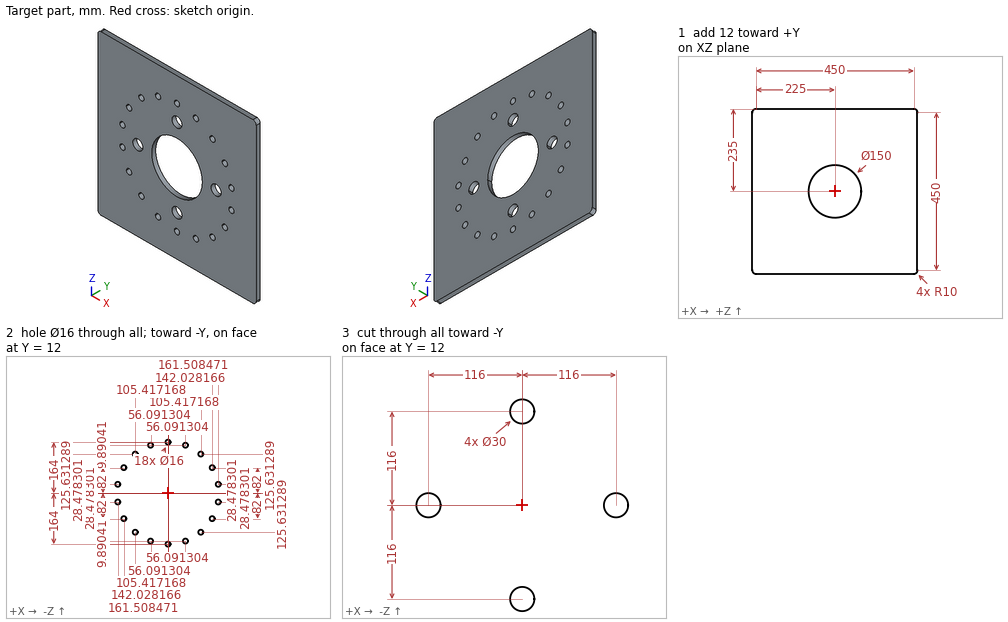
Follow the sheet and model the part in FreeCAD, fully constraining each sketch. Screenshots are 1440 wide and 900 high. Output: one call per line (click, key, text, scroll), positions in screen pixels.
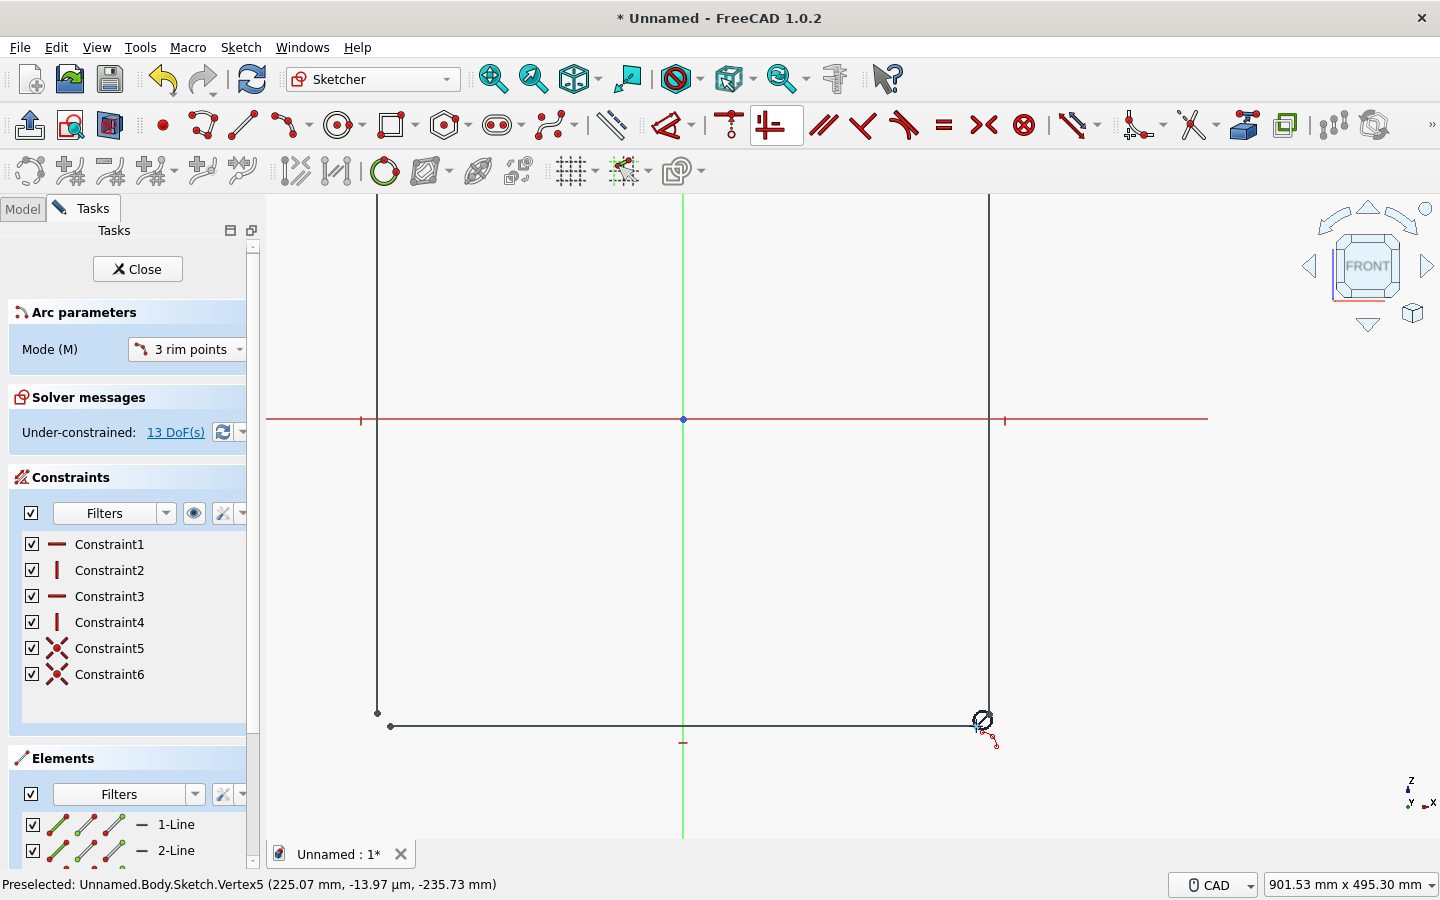
scroll(985, 722, up, 8)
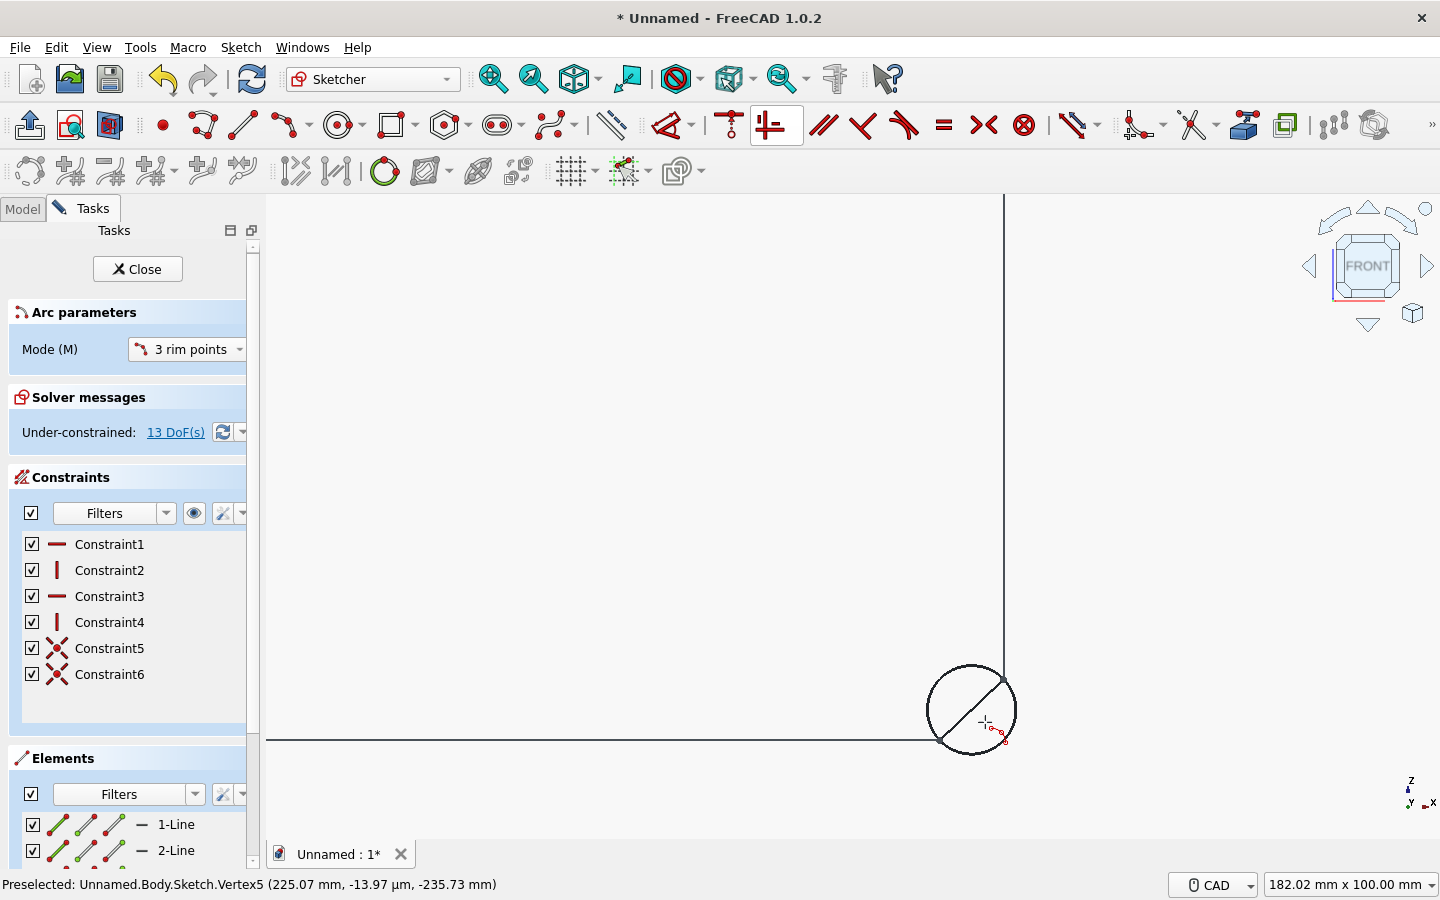
click(985, 717)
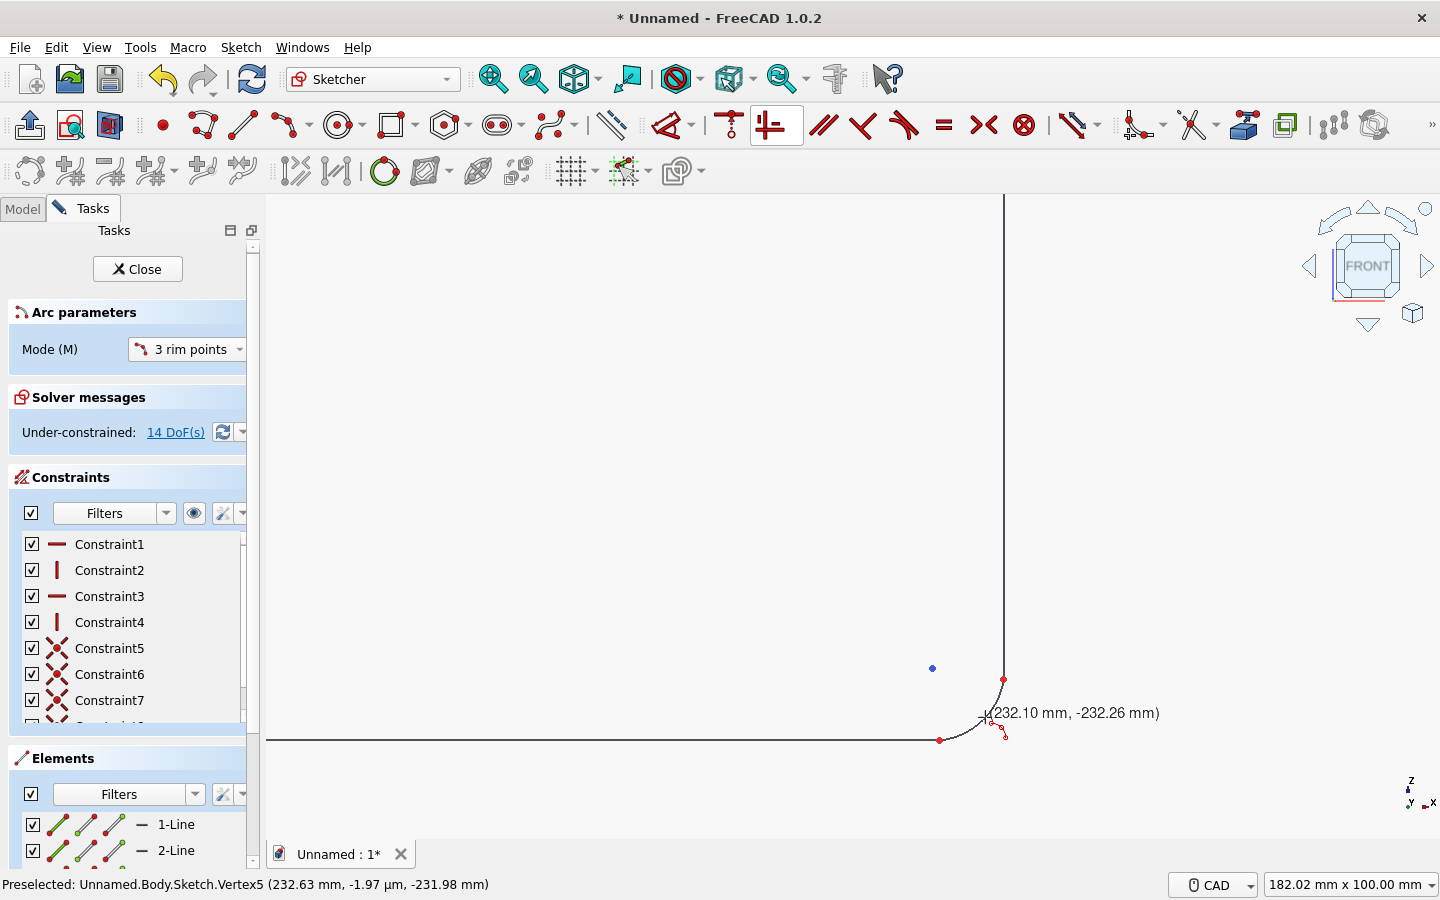
scroll(987, 719, down, 10)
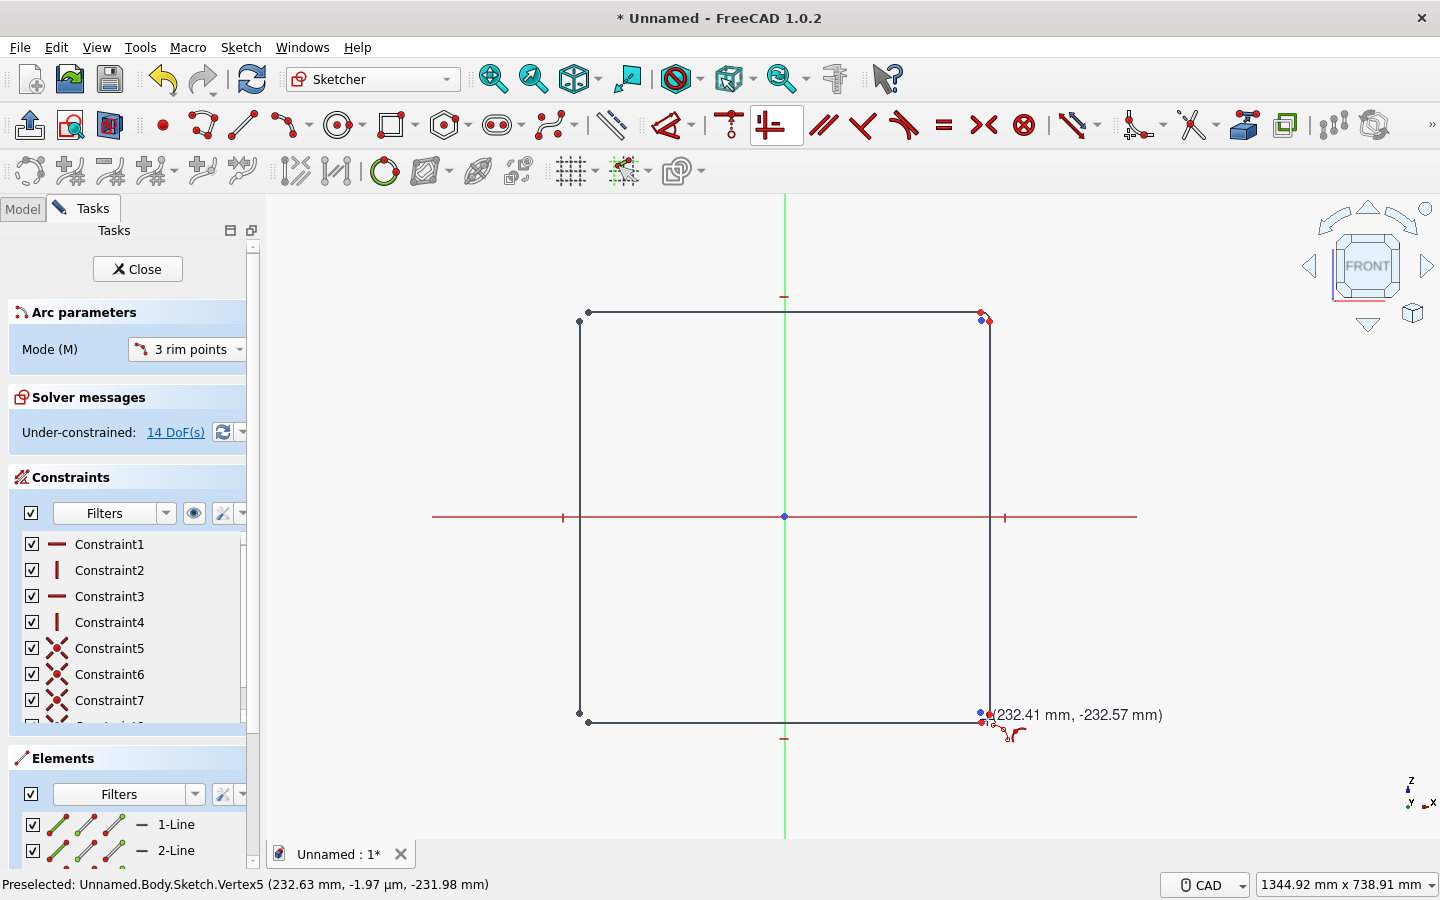
scroll(588, 722, up, 2)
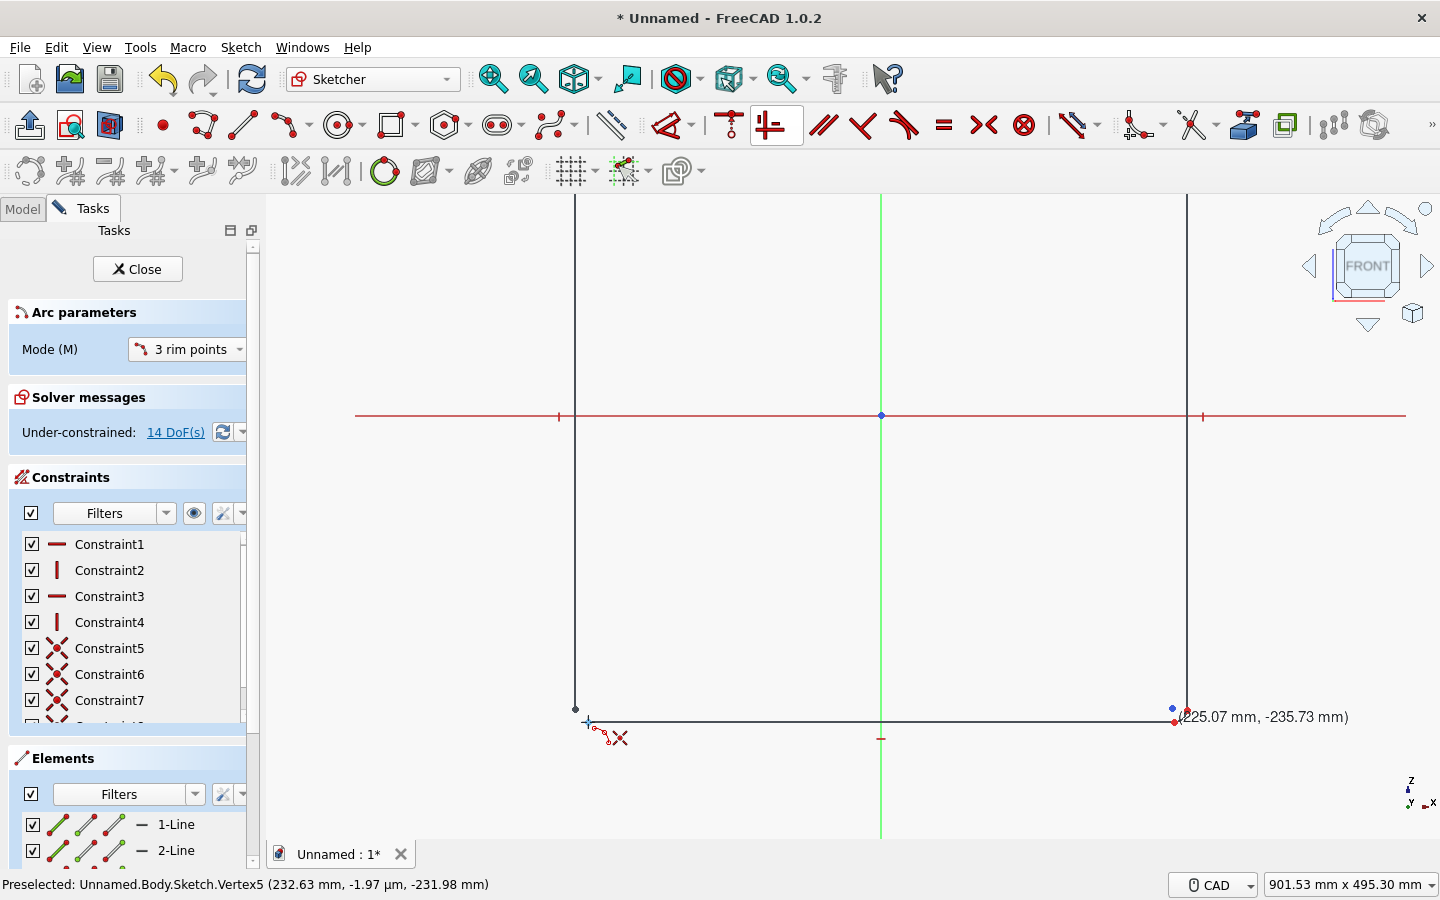
click(588, 722)
click(575, 709)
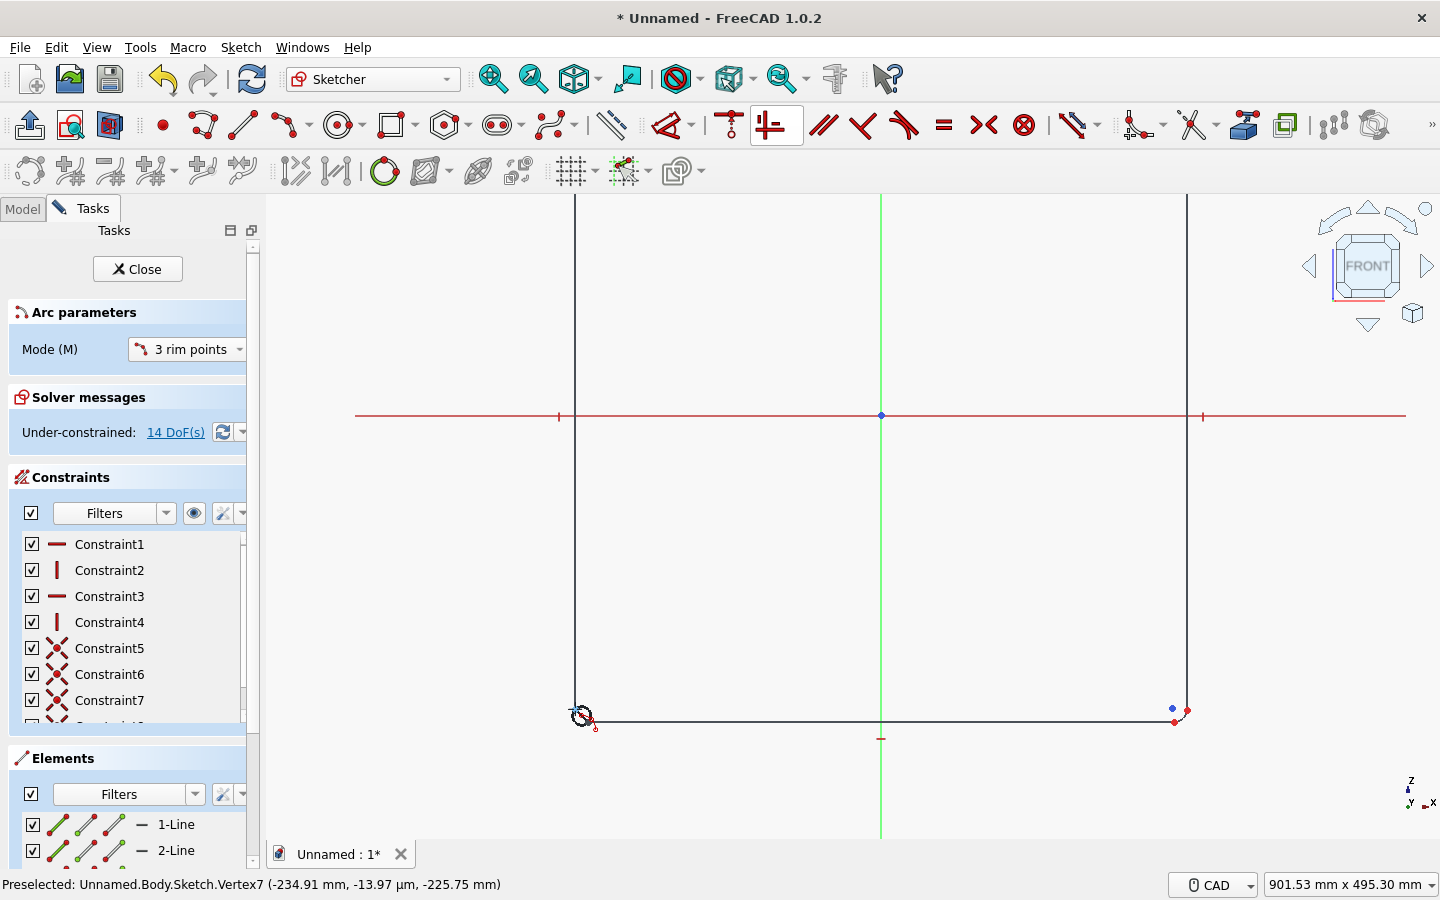
scroll(579, 718, up, 8)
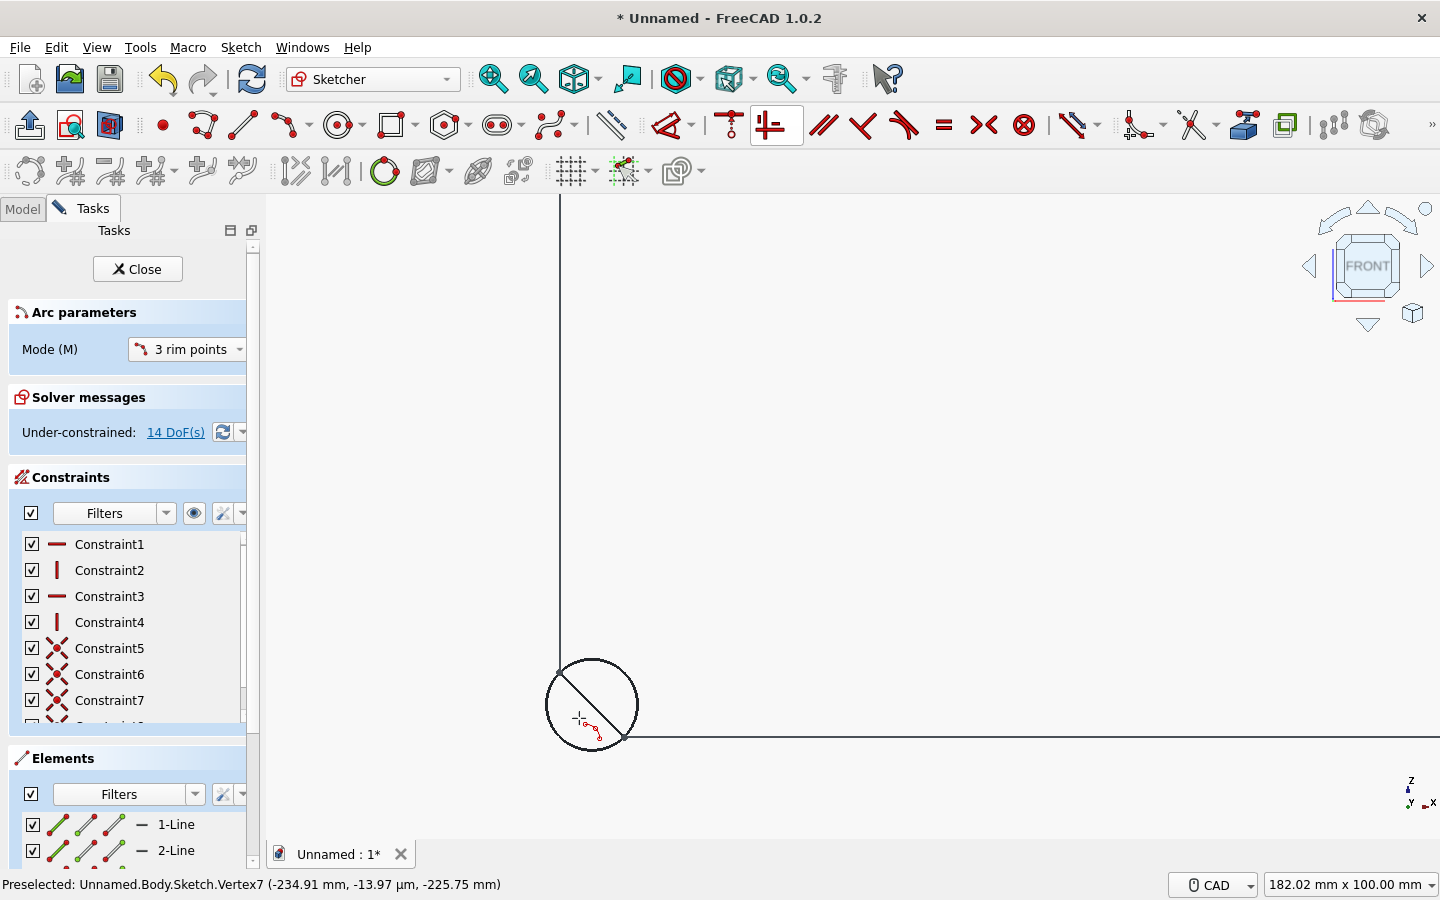
click(578, 713)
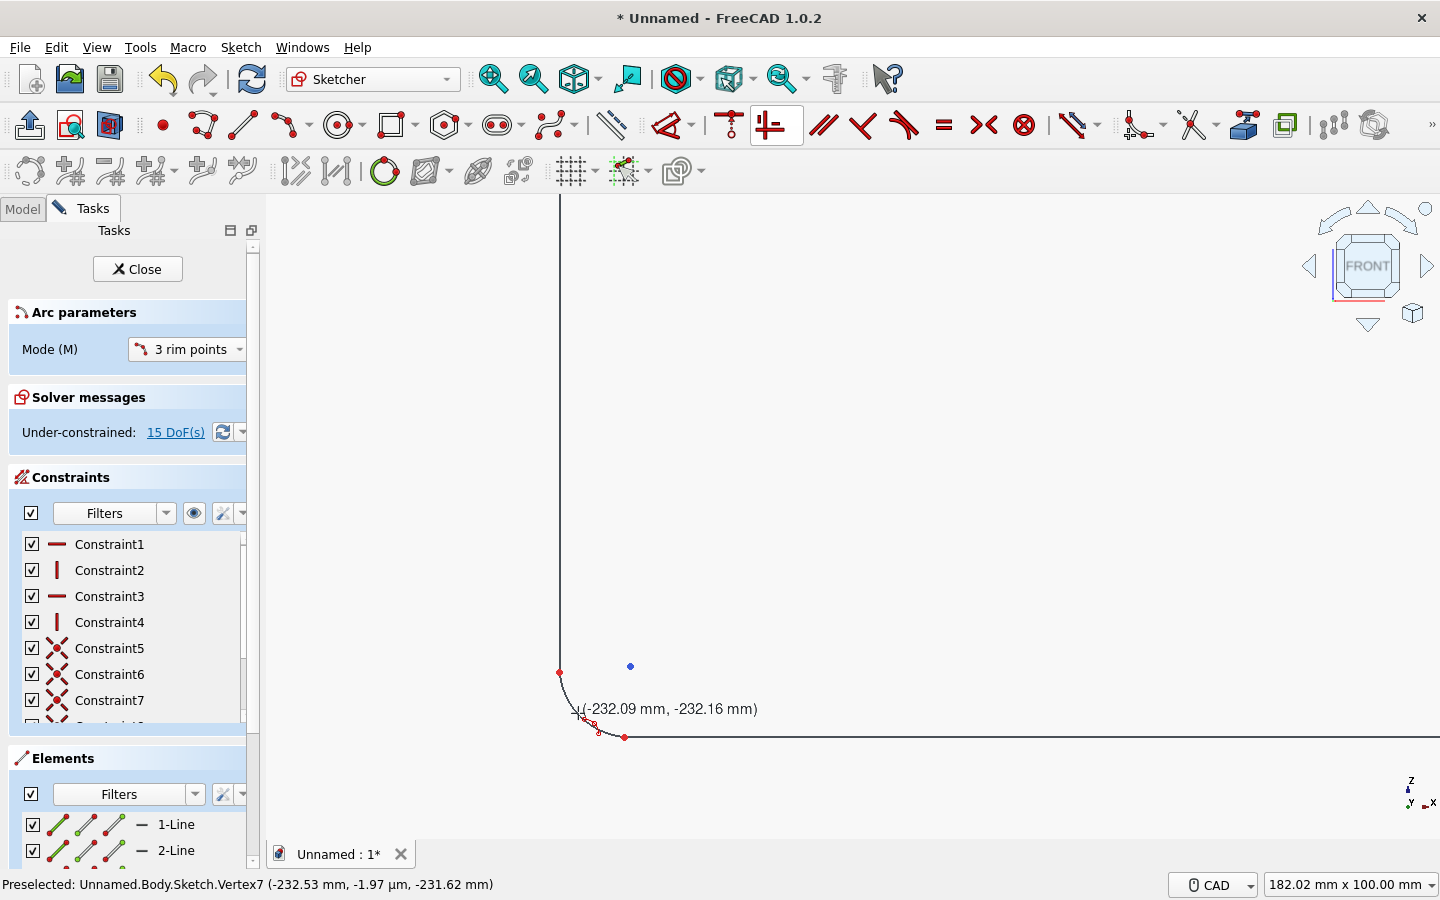
scroll(583, 720, down, 10)